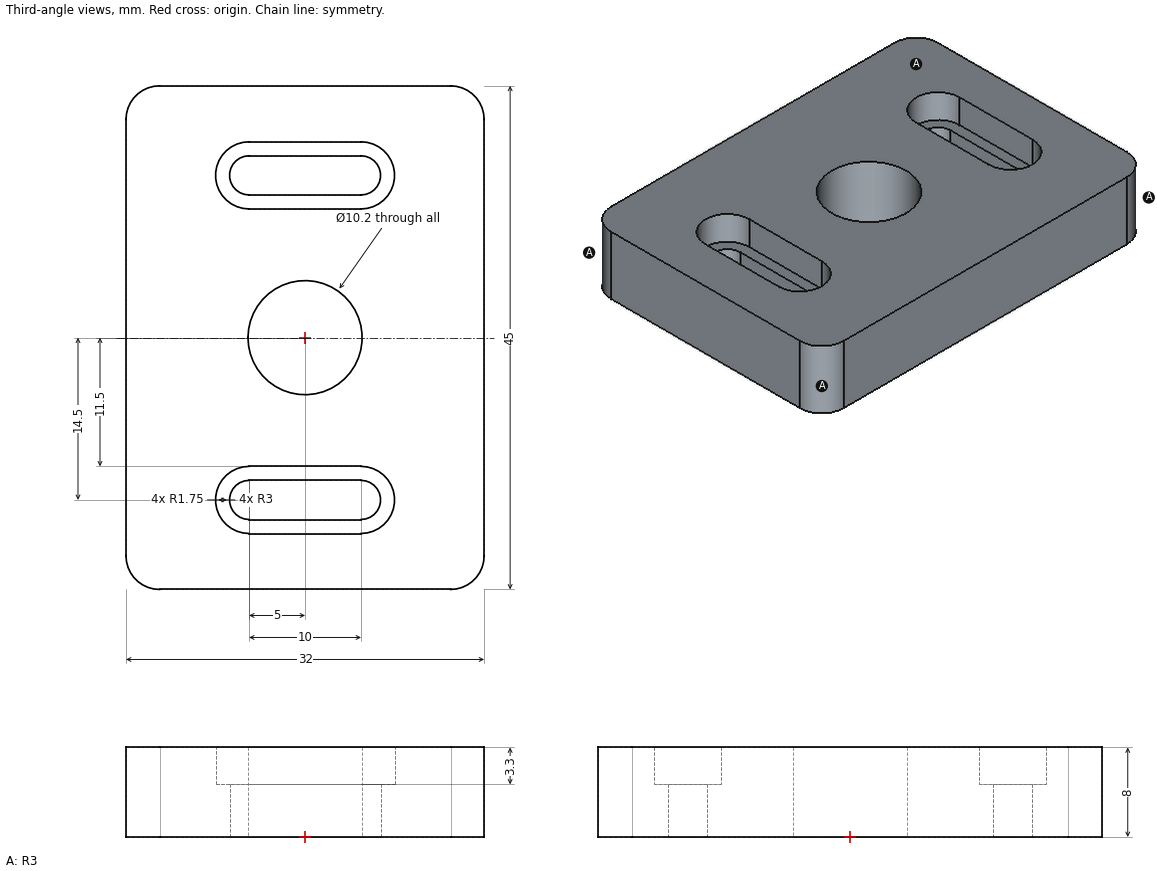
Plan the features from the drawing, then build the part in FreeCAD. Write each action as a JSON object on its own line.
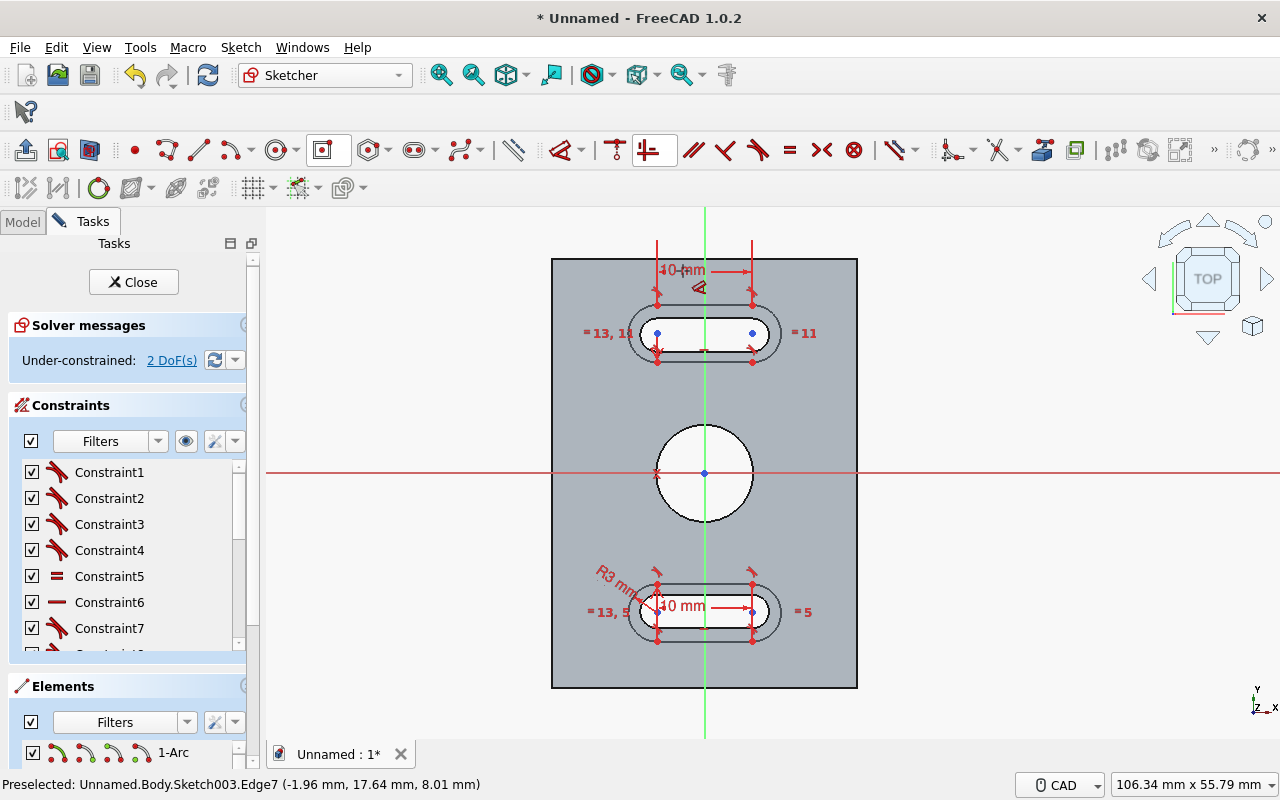
{"action": "left_click", "coordinate": [657, 584]}
{"action": "left_click", "coordinate": [681, 439]}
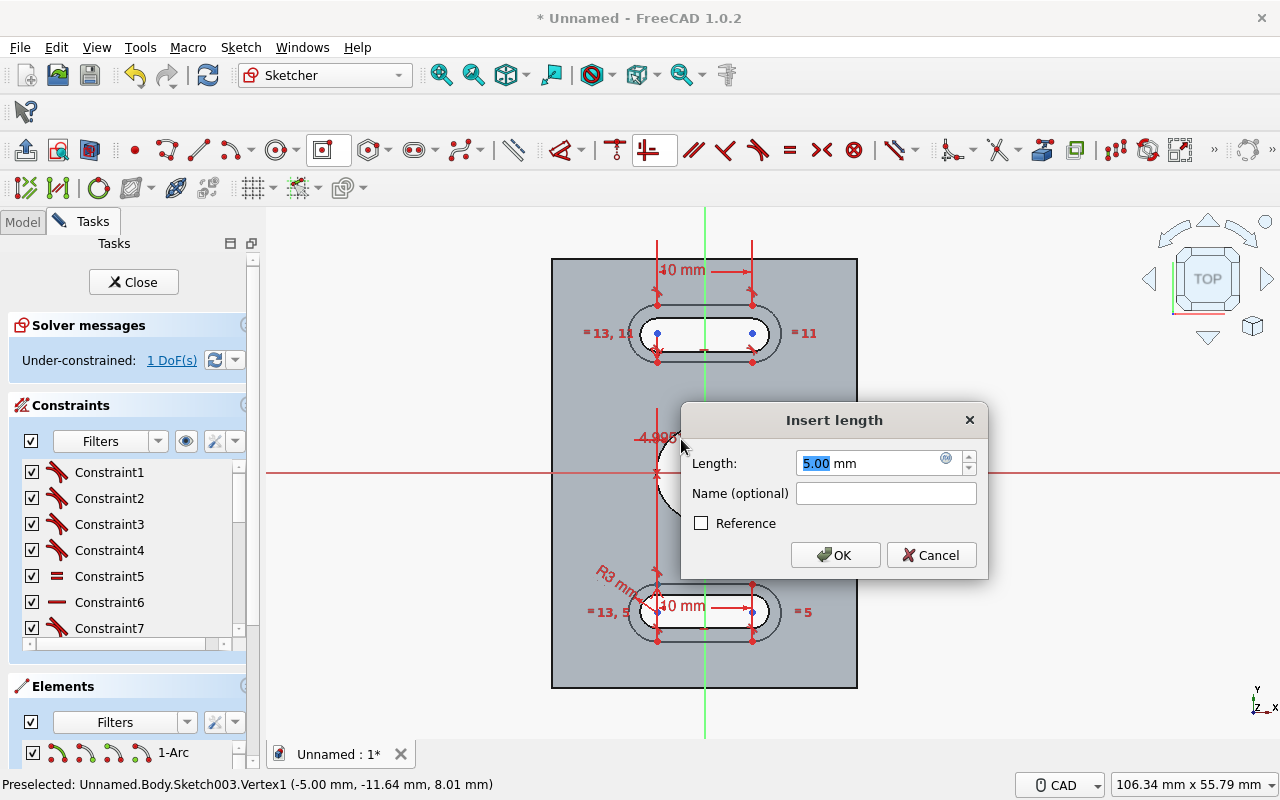
{"action": "type", "text": "5"}
{"action": "key", "text": "Return"}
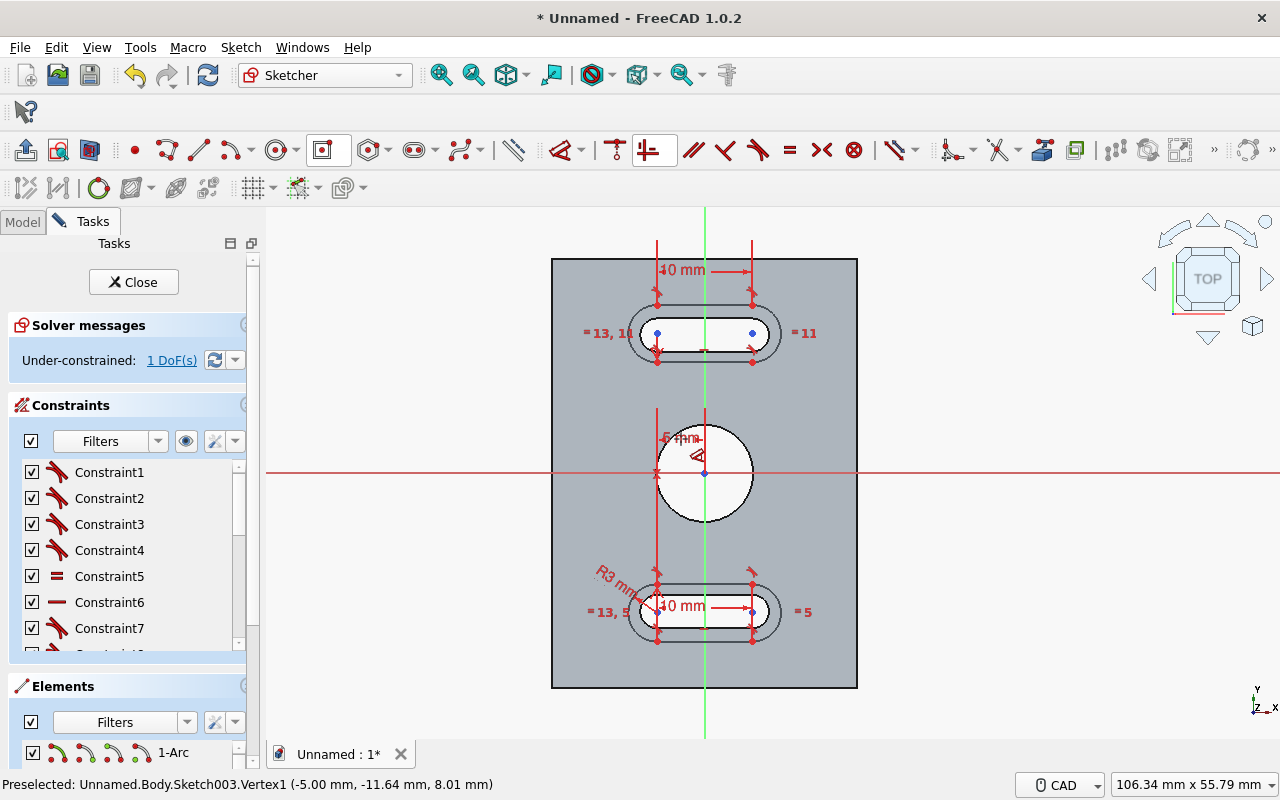
{"action": "left_click", "coordinate": [657, 584]}
{"action": "left_click", "coordinate": [623, 529]}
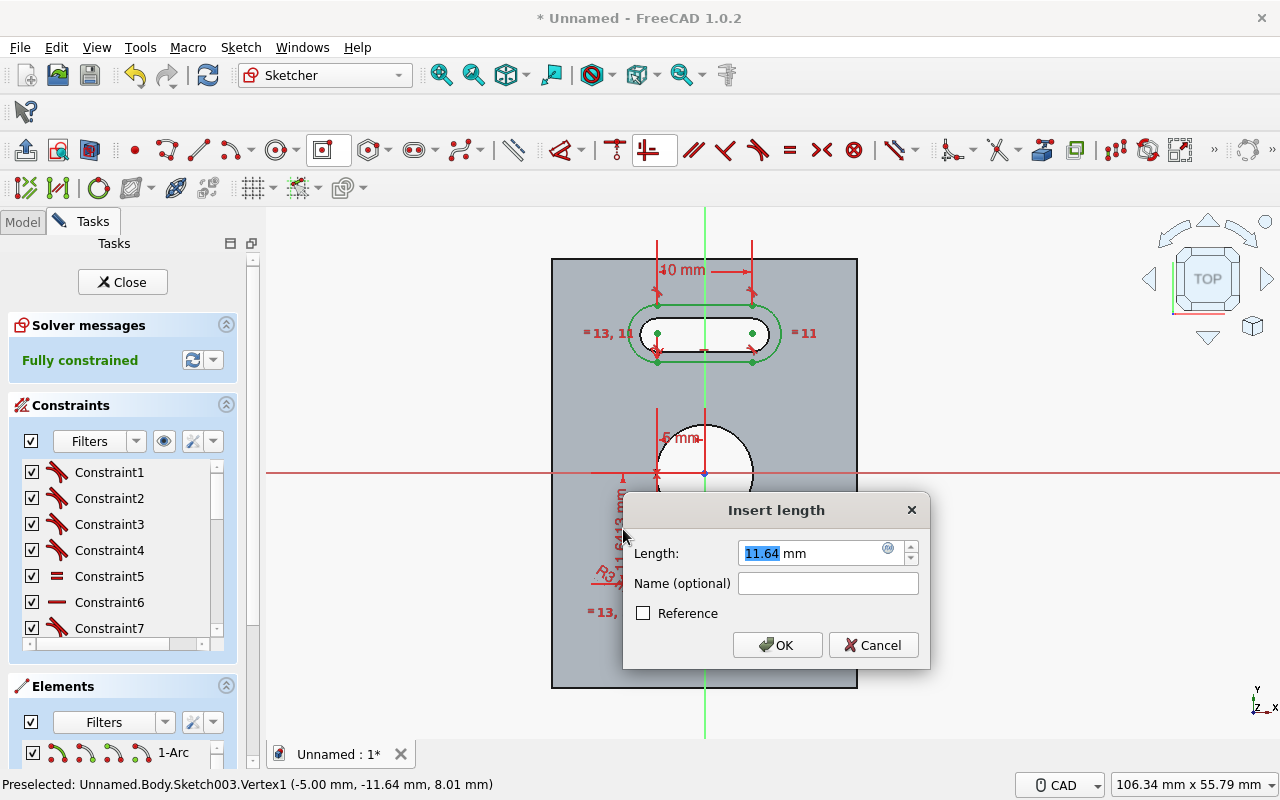
{"action": "type", "text": "11.5"}
{"action": "key", "text": "Return"}
{"action": "key", "text": "Escape"}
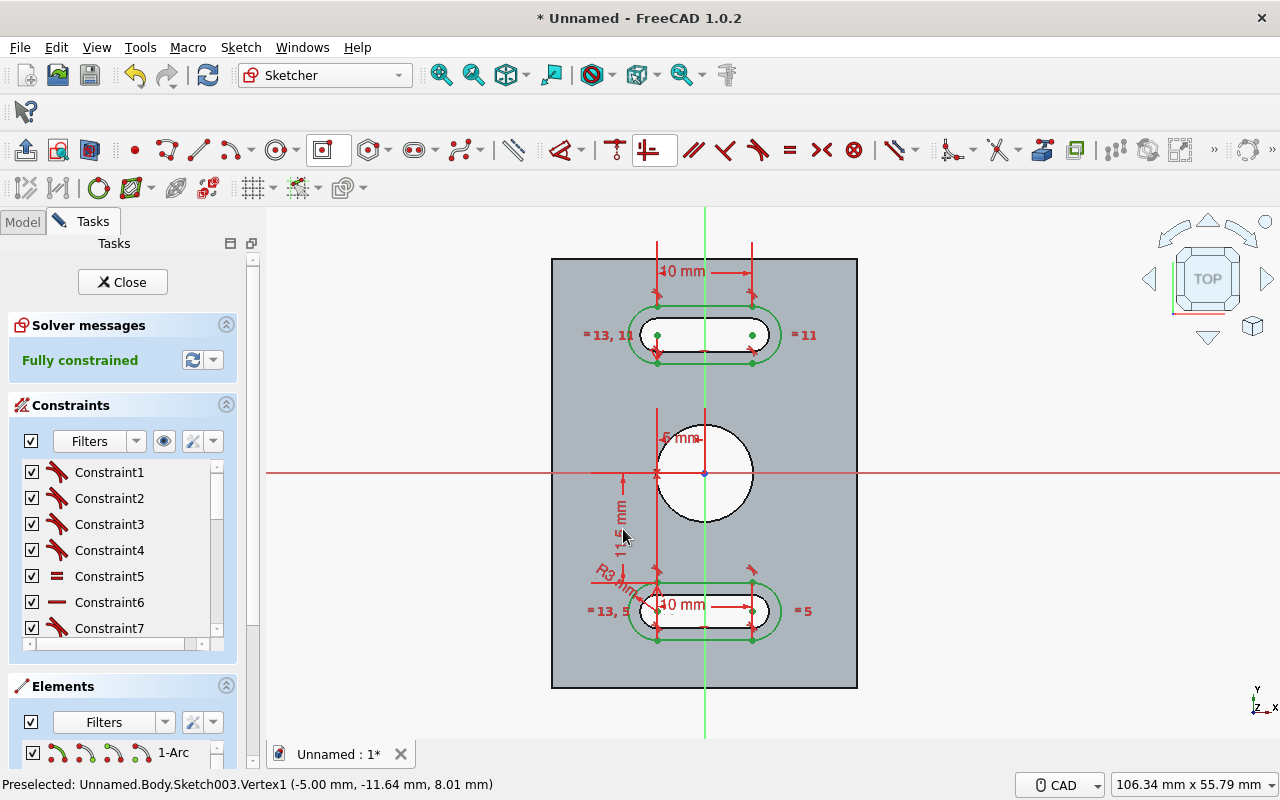
{"action": "left_click", "coordinate": [123, 282]}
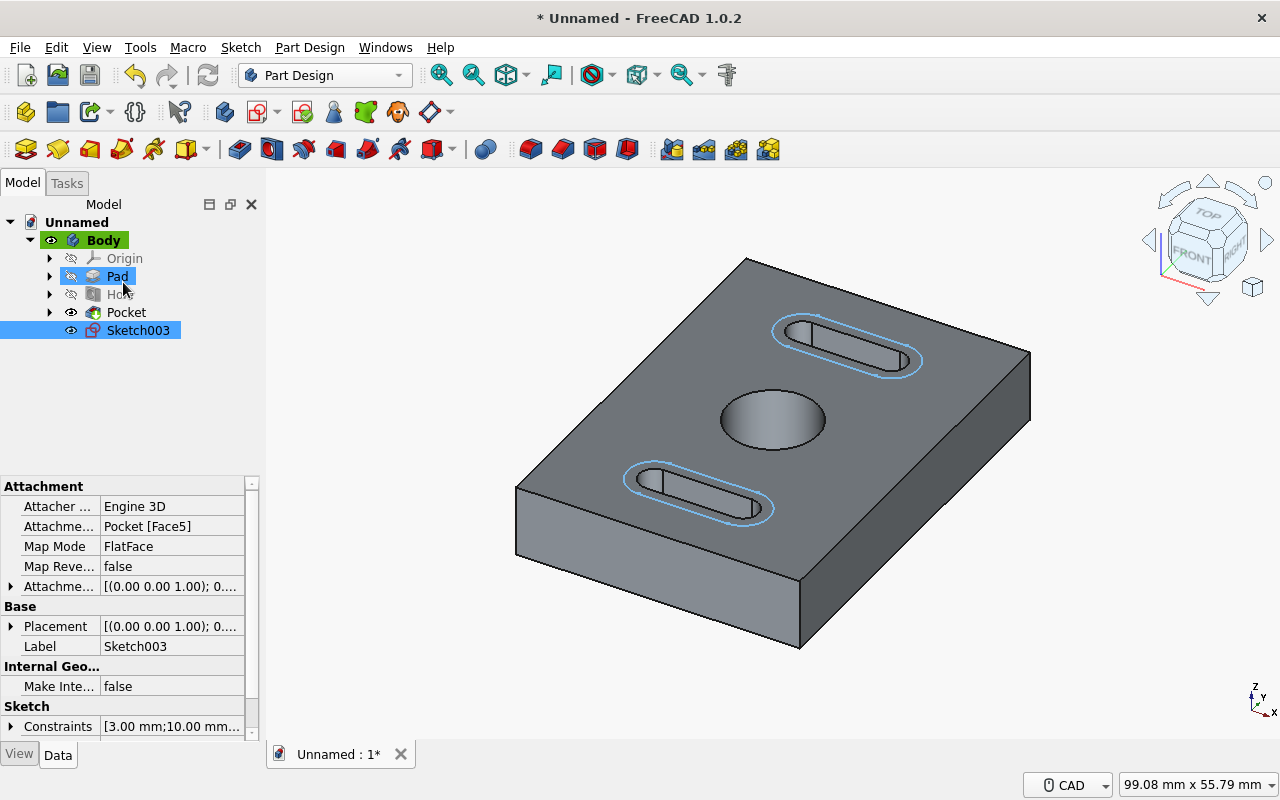
{"action": "left_click", "coordinate": [240, 150]}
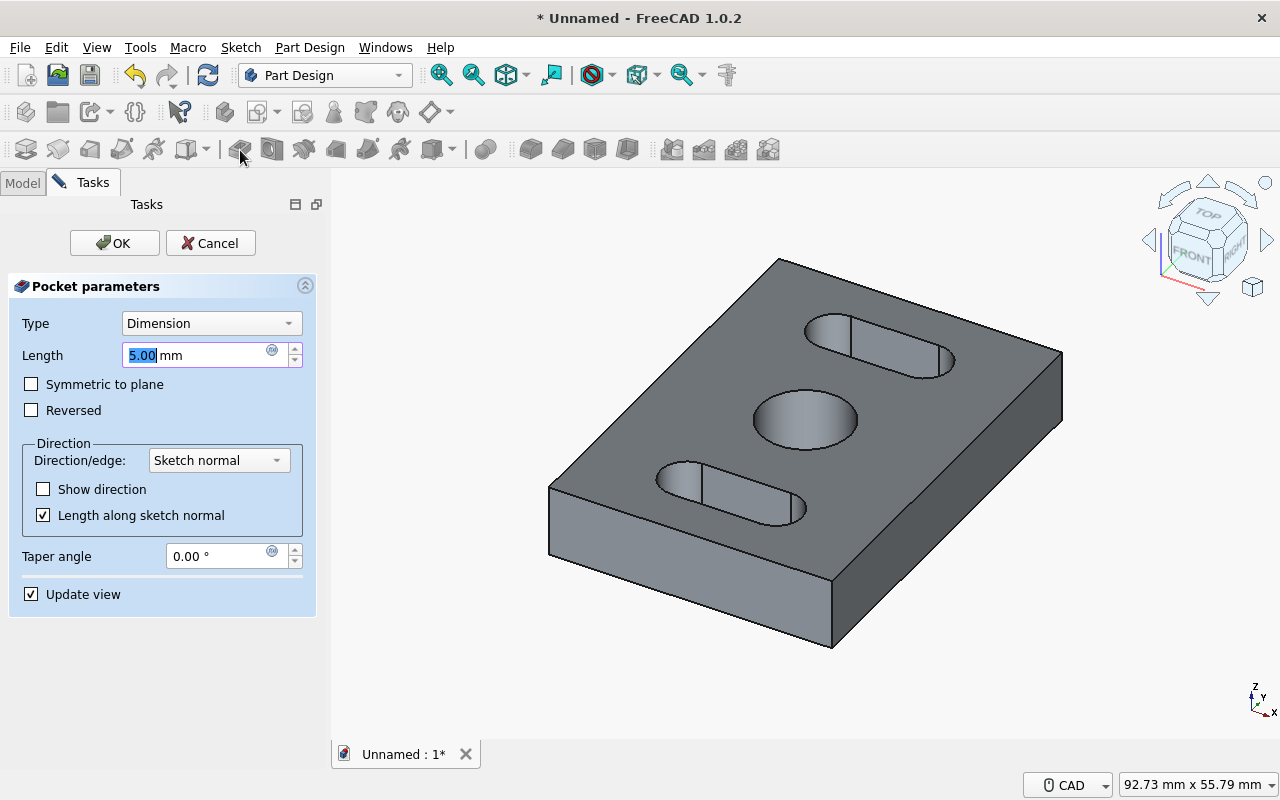
{"action": "type", "text": "3.3"}
{"action": "key", "text": "Tab"}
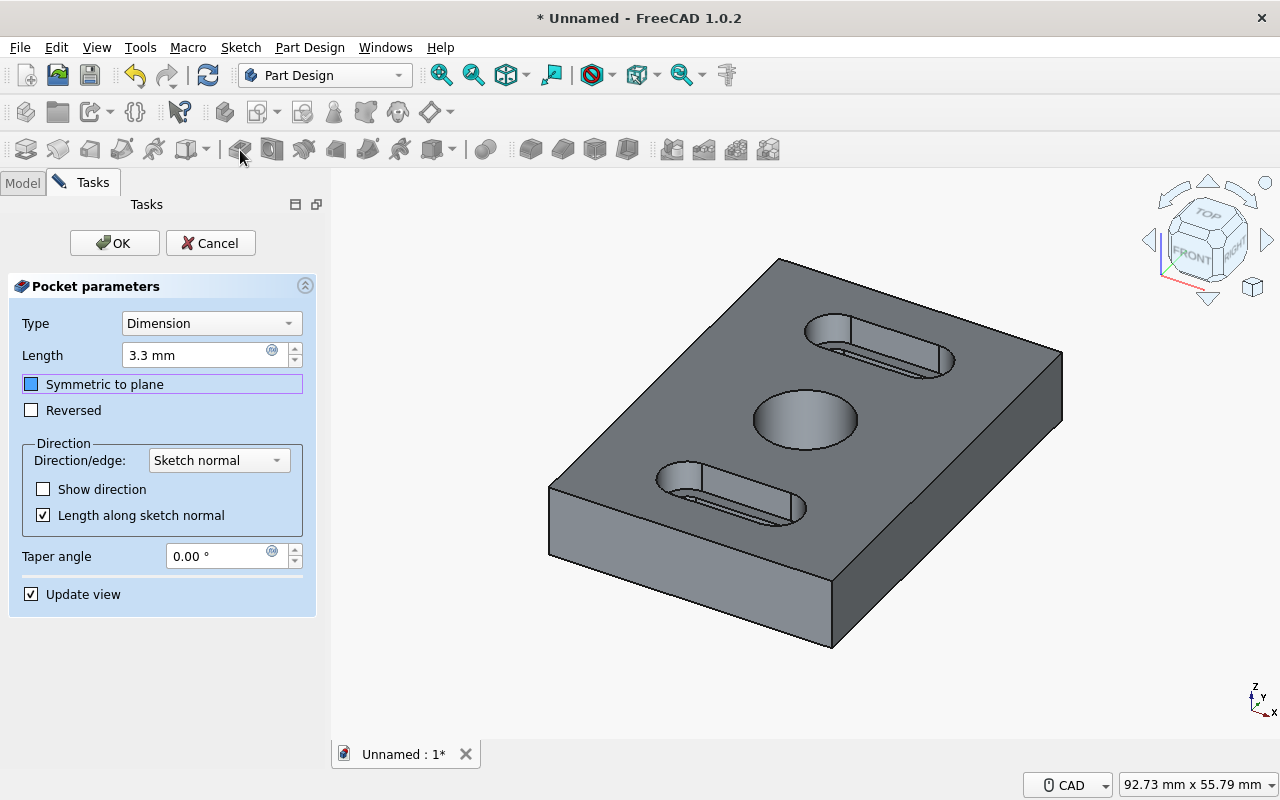
{"action": "left_click", "coordinate": [115, 243]}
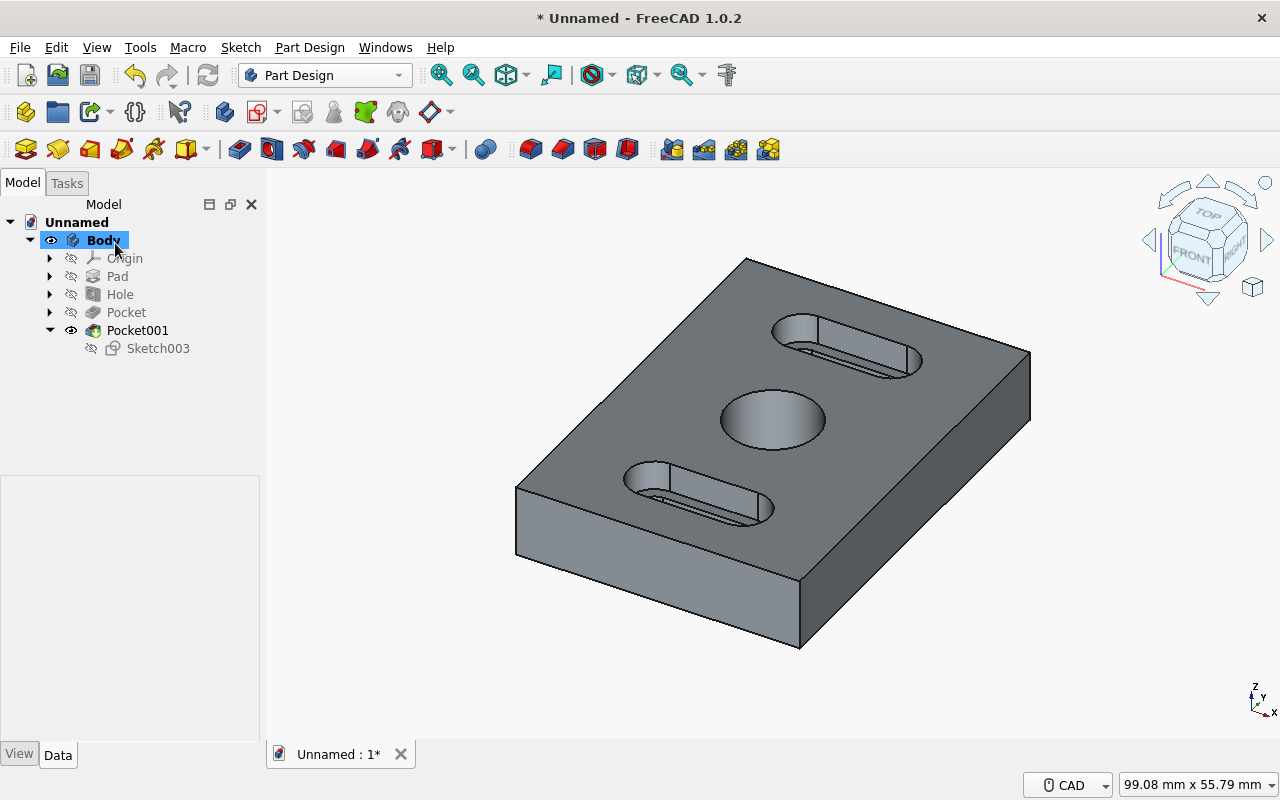
{"action": "left_click", "coordinate": [800, 614]}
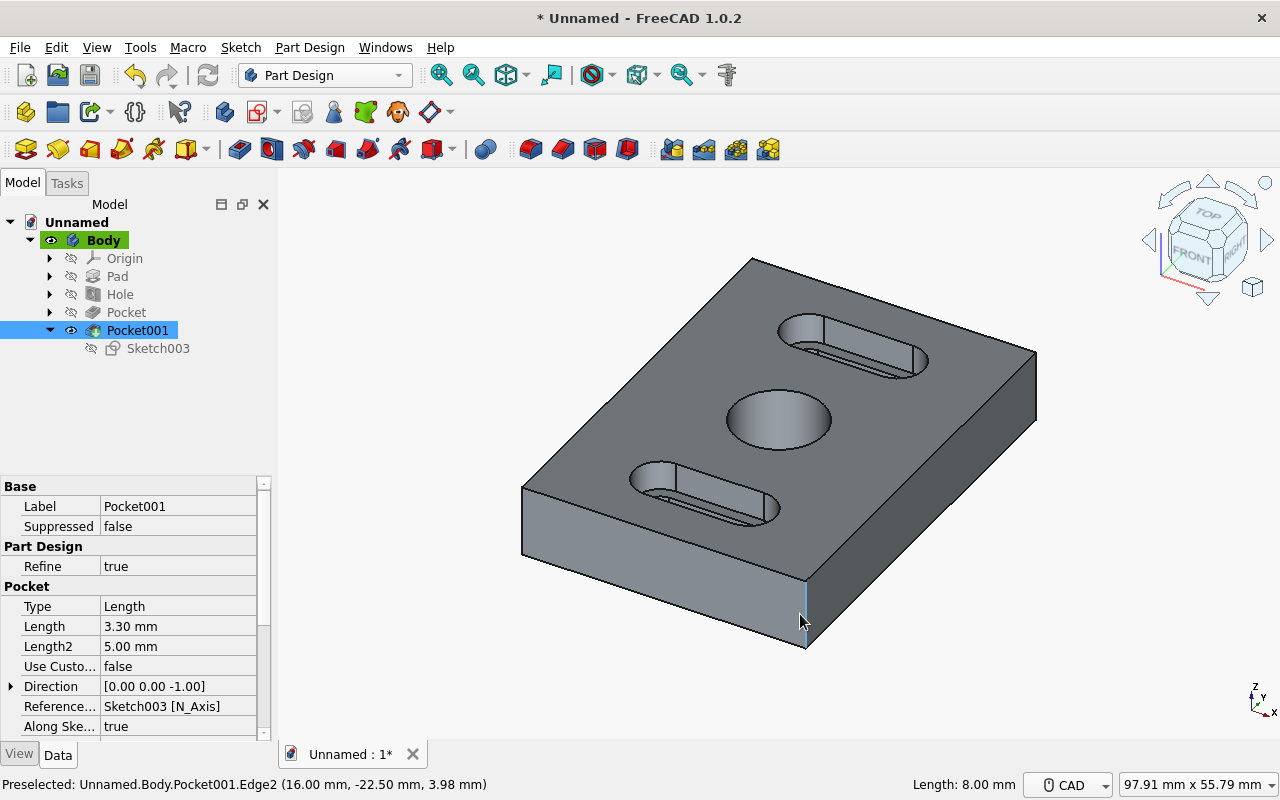
{"action": "key", "text": "0"}